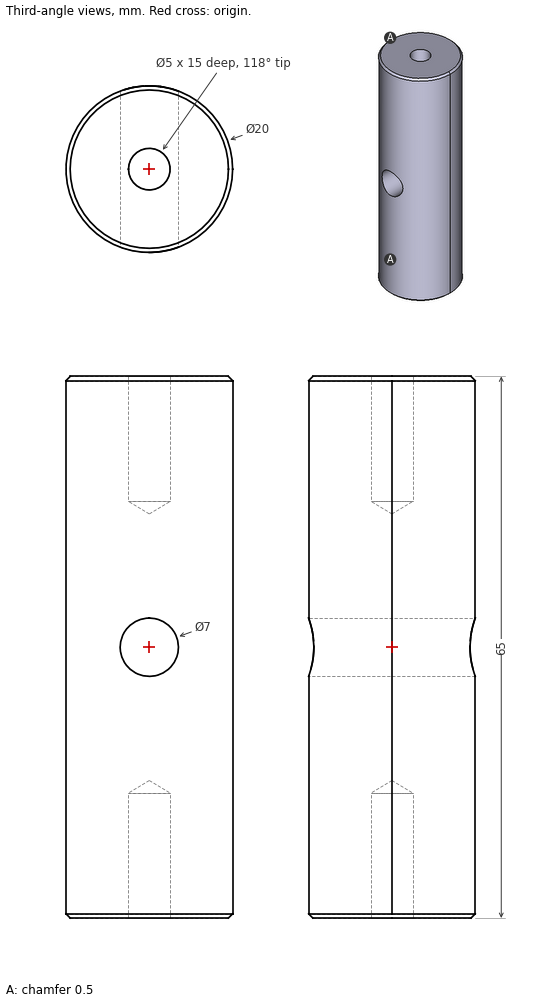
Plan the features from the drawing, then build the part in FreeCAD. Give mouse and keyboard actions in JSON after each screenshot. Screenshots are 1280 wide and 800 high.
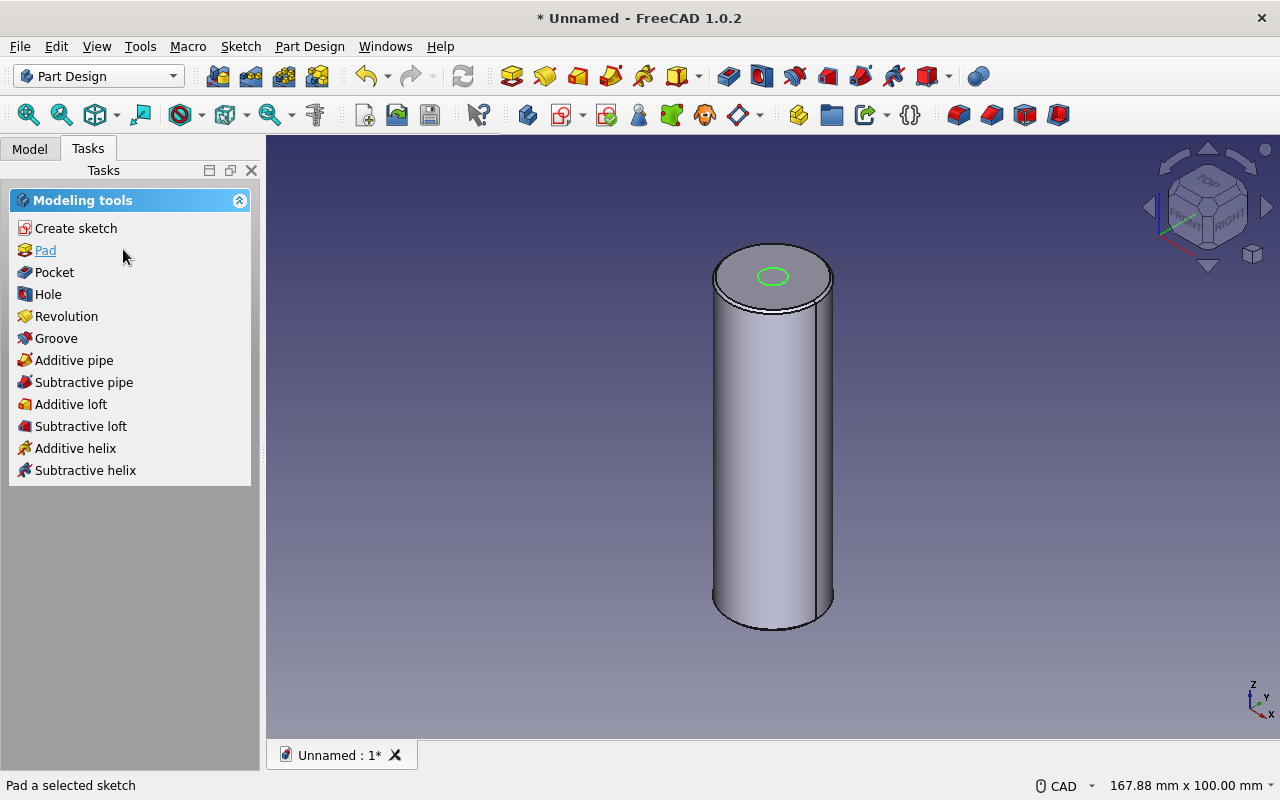
{"action": "left_click", "coordinate": [762, 76]}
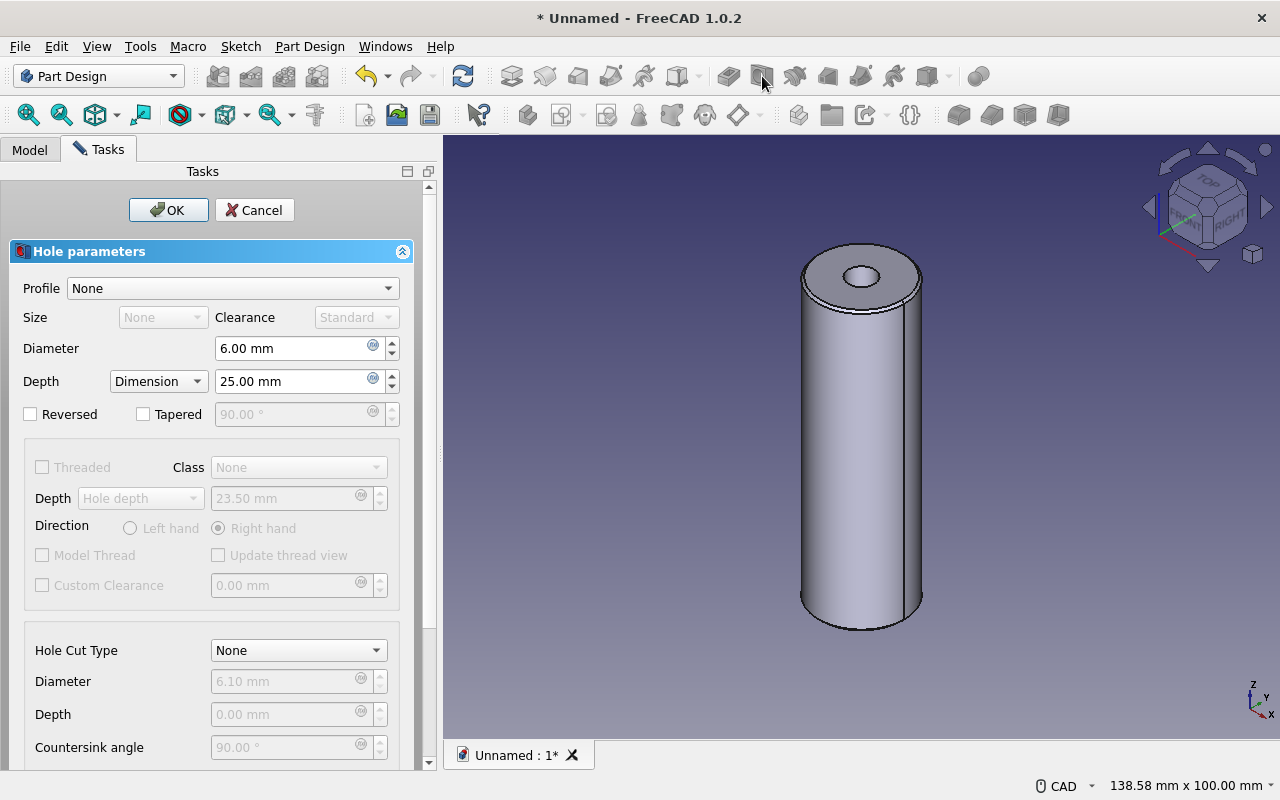
{"action": "triple_click", "coordinate": [300, 348]}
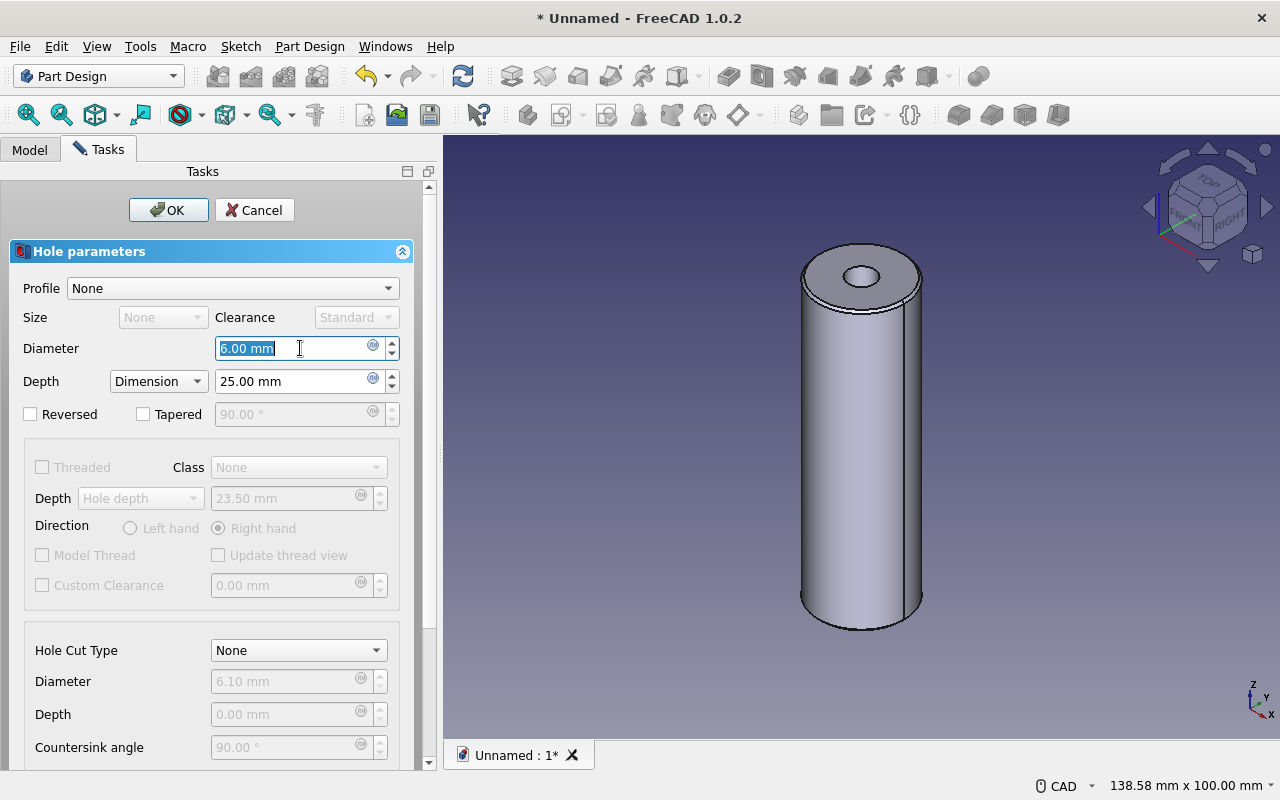
{"action": "type", "text": "5"}
{"action": "key", "text": "Tab"}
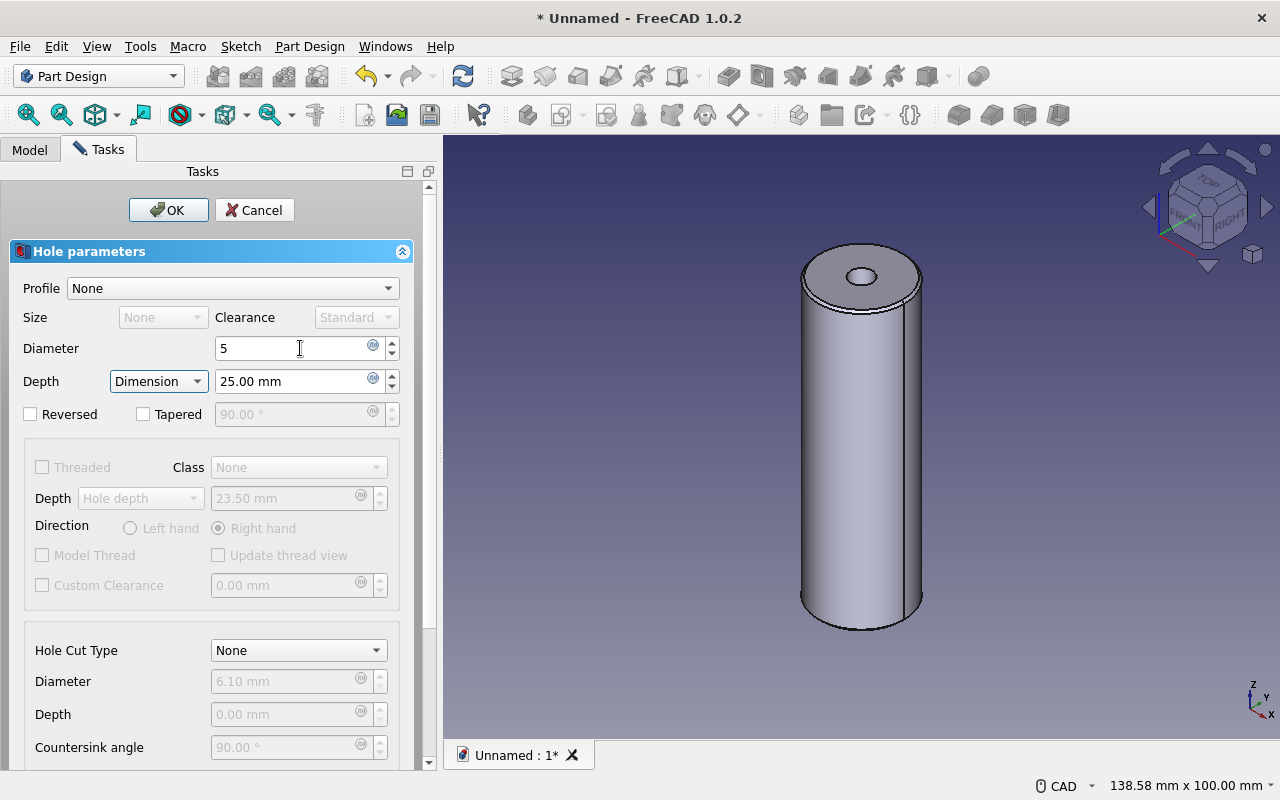
{"action": "triple_click", "coordinate": [300, 382]}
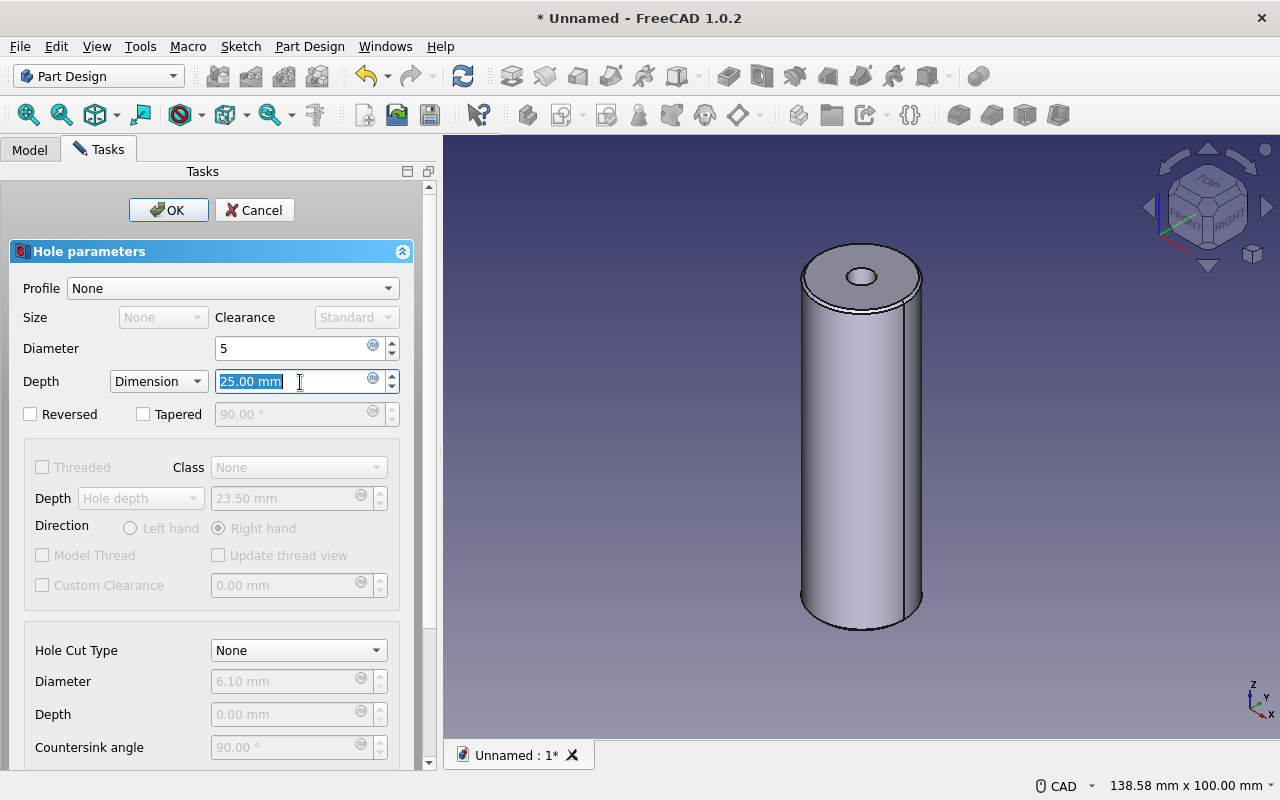
{"action": "type", "text": "15"}
{"action": "key", "text": "Tab"}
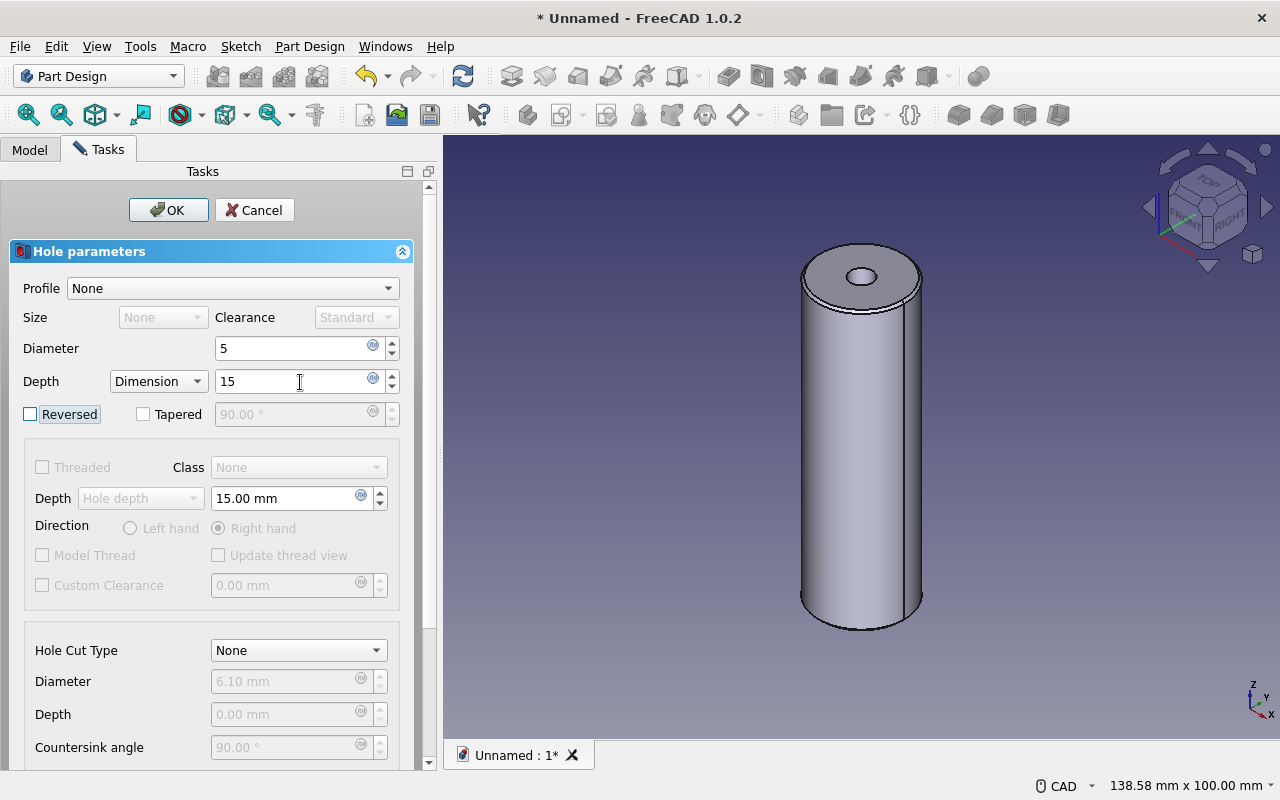
{"action": "left_click", "coordinate": [169, 210]}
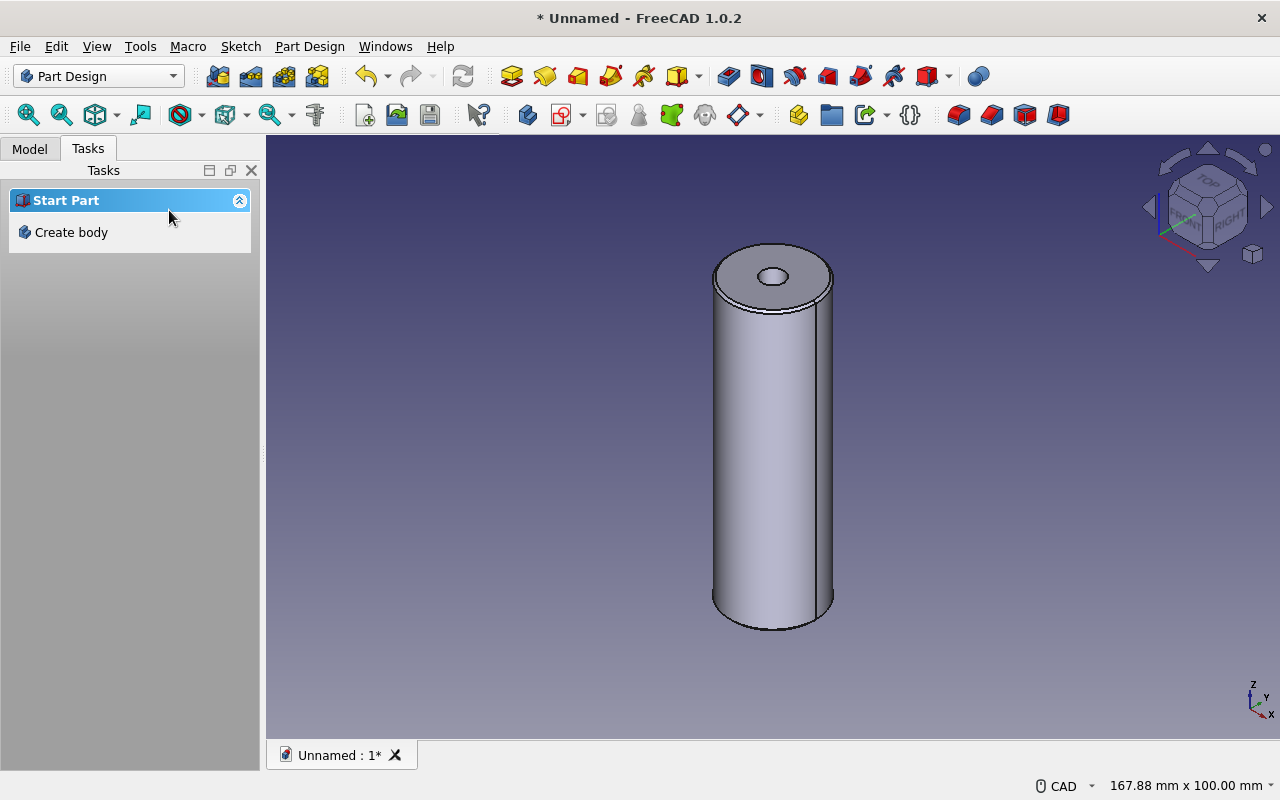
{"action": "key", "text": "5"}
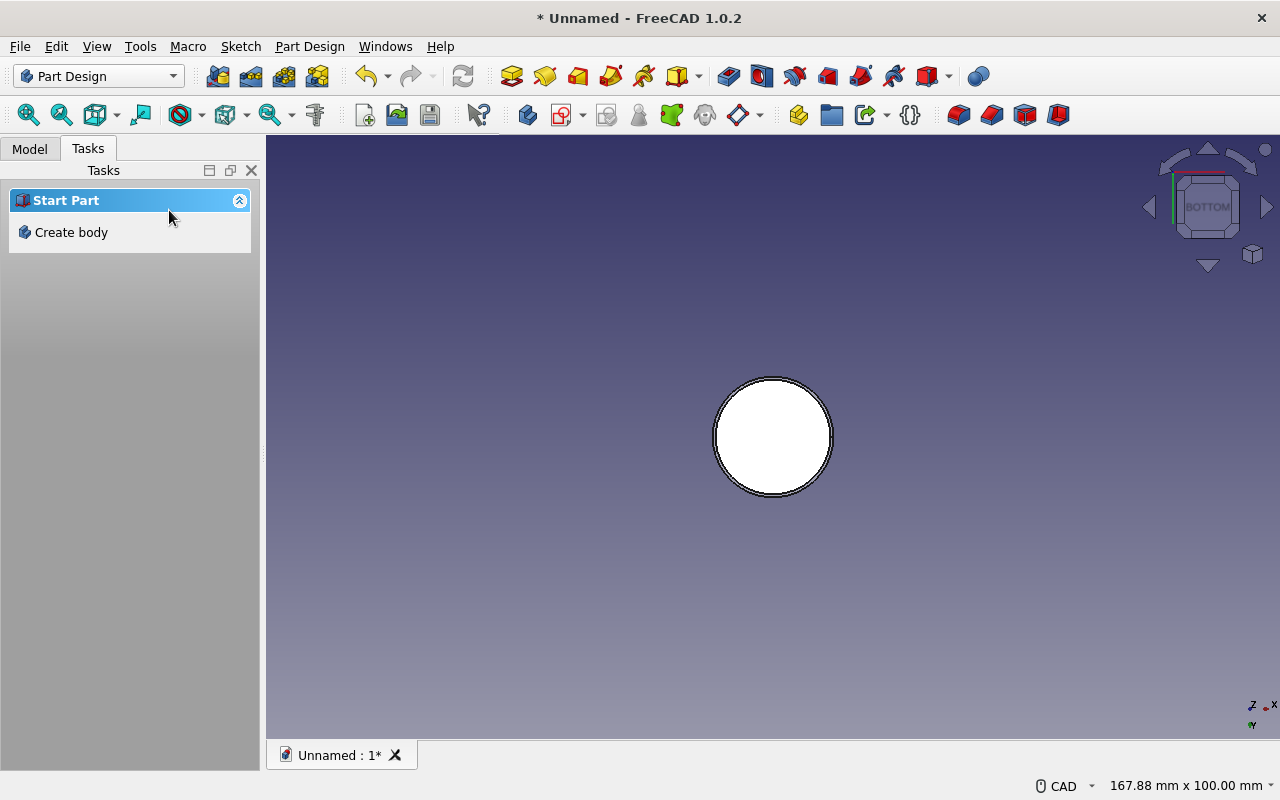
{"action": "left_click", "coordinate": [29, 116]}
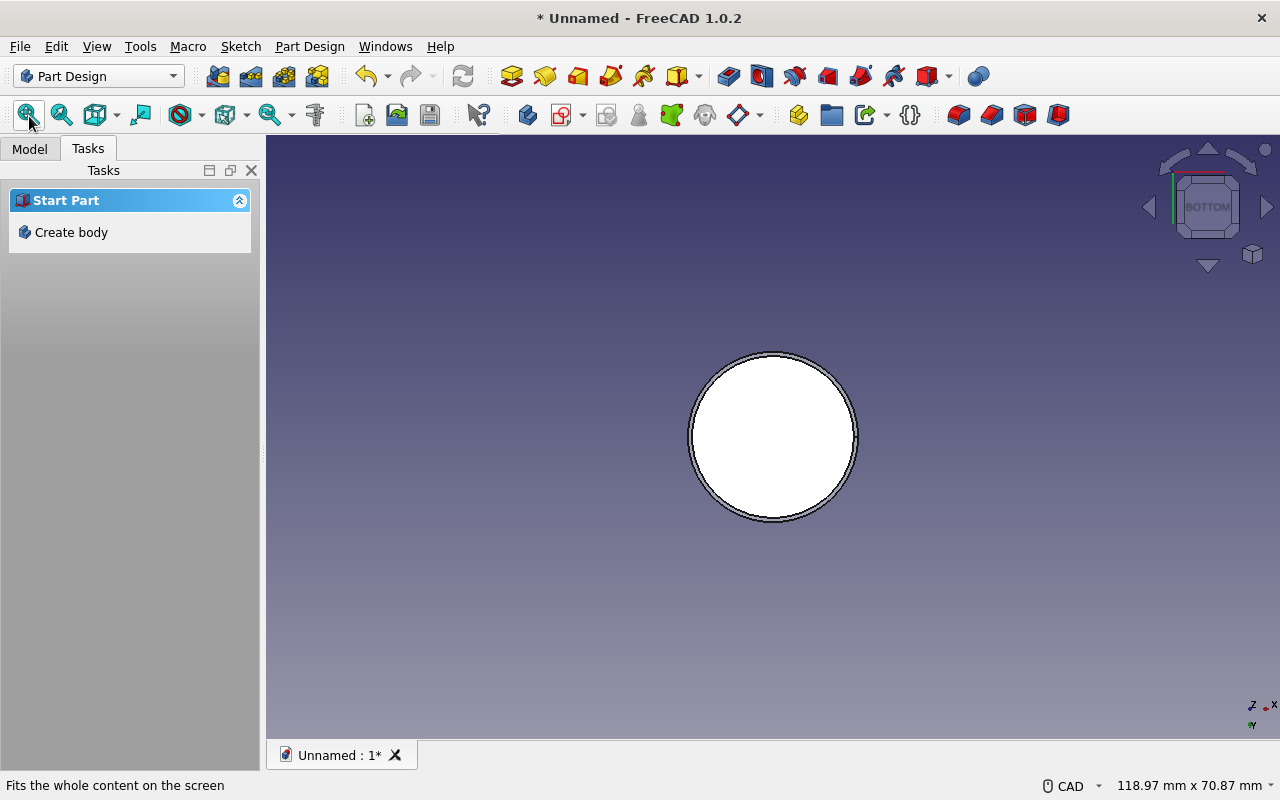
{"action": "left_click", "coordinate": [773, 436]}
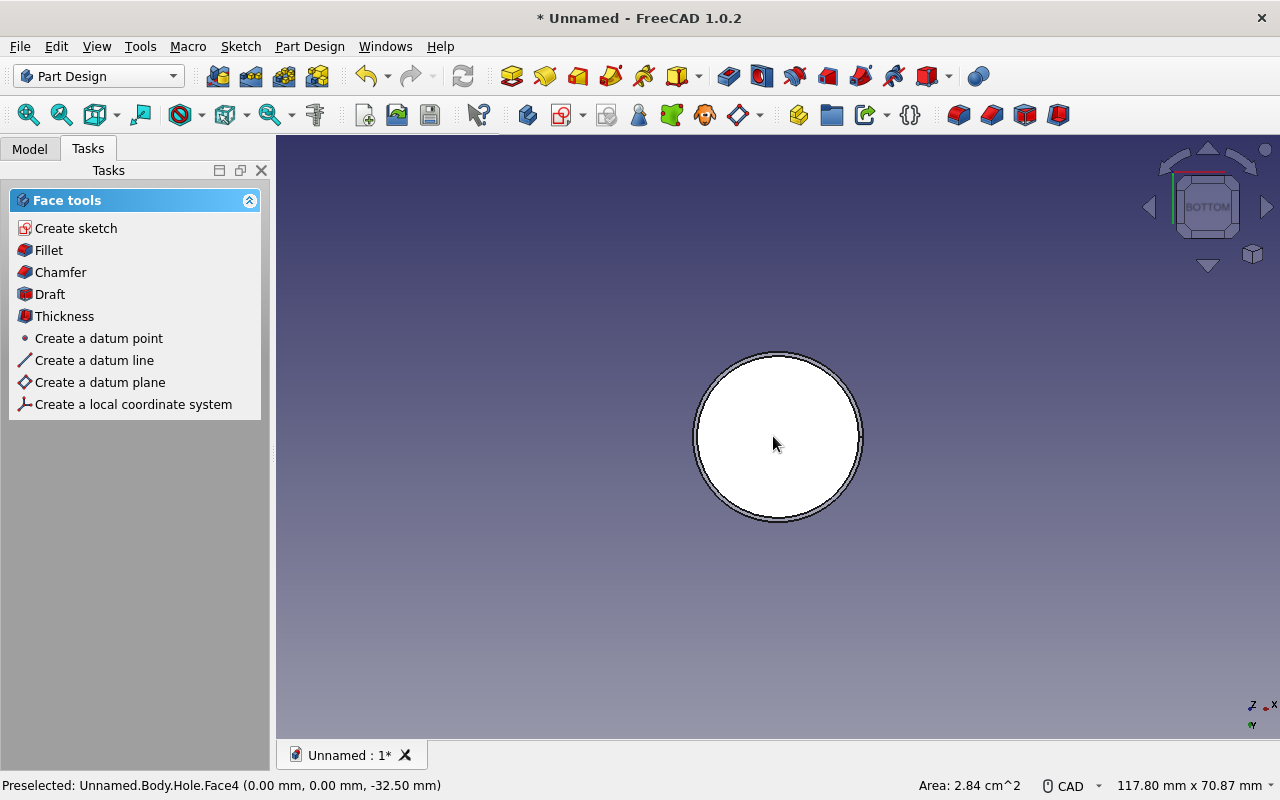
{"action": "left_click", "coordinate": [560, 116]}